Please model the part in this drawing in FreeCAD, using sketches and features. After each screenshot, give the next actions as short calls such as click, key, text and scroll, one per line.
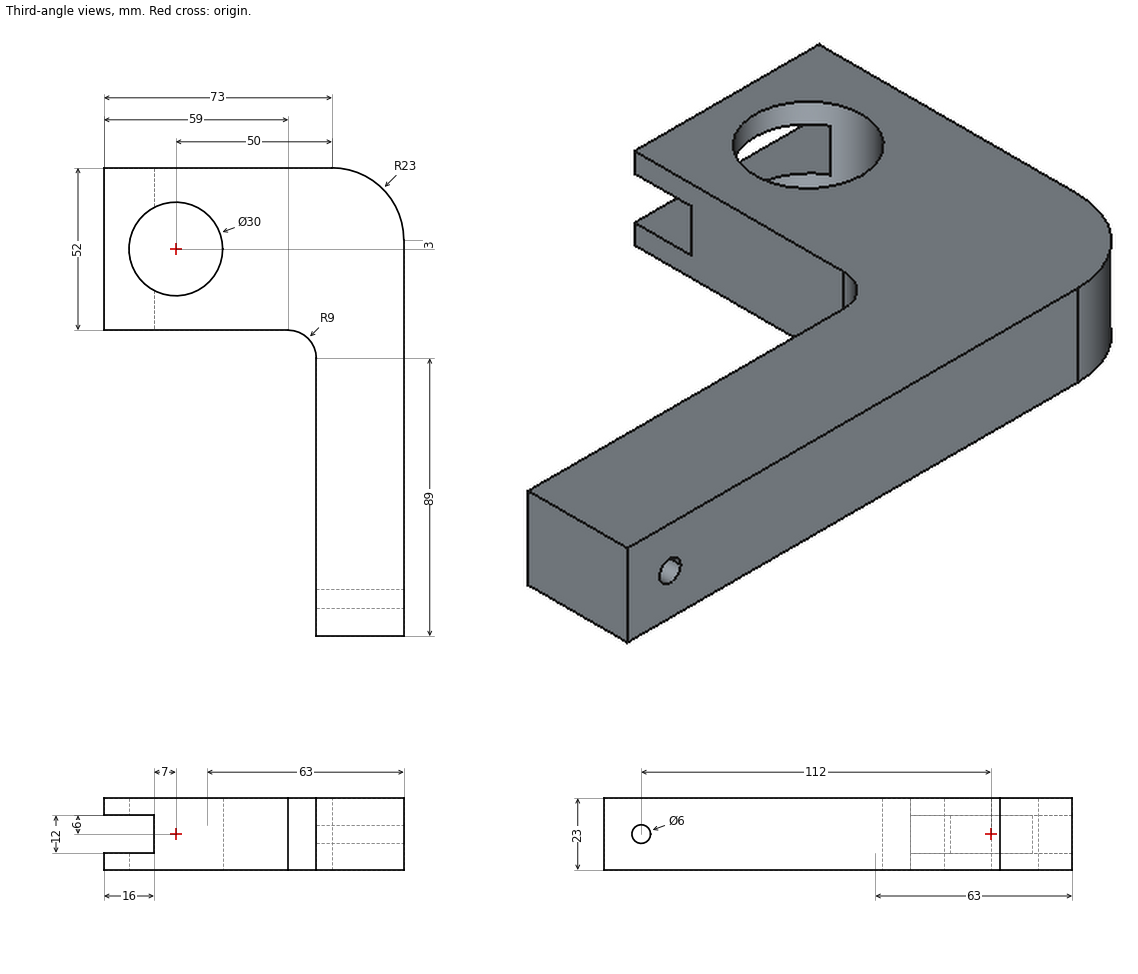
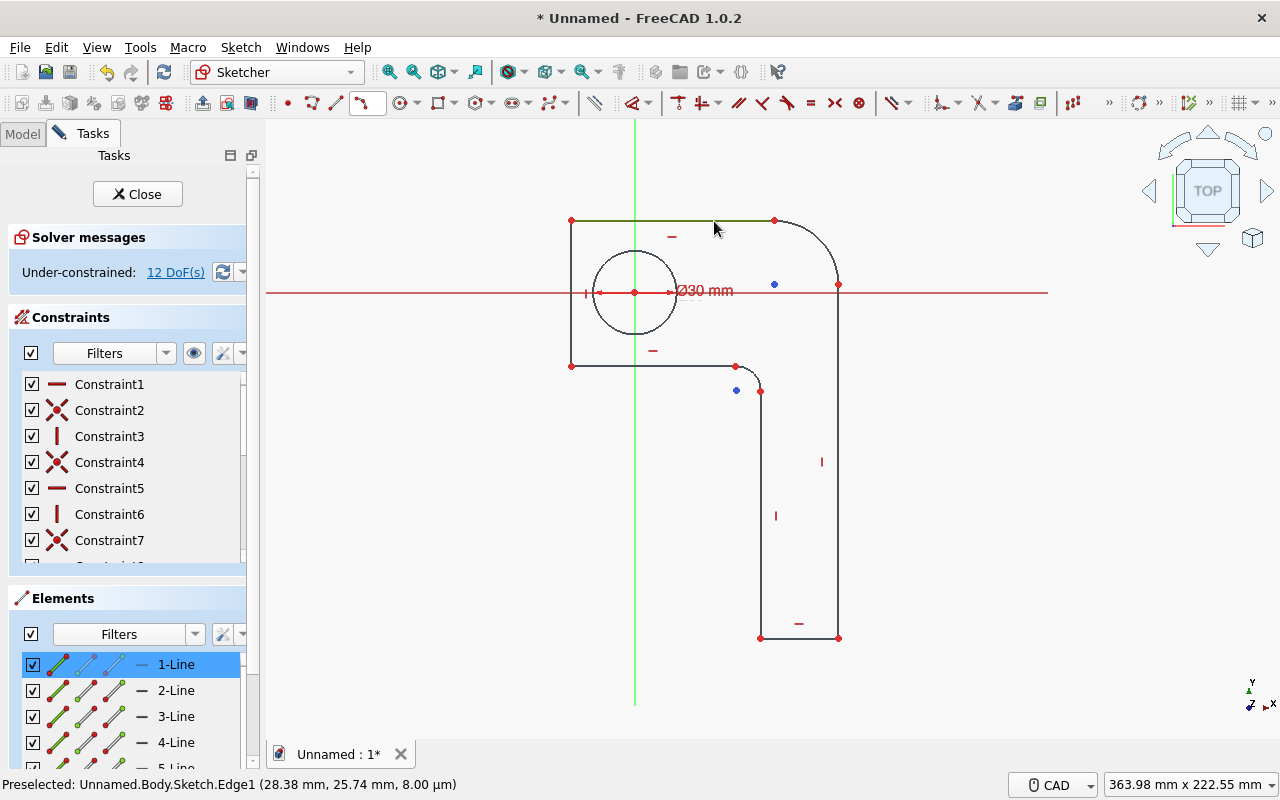
click(831, 256)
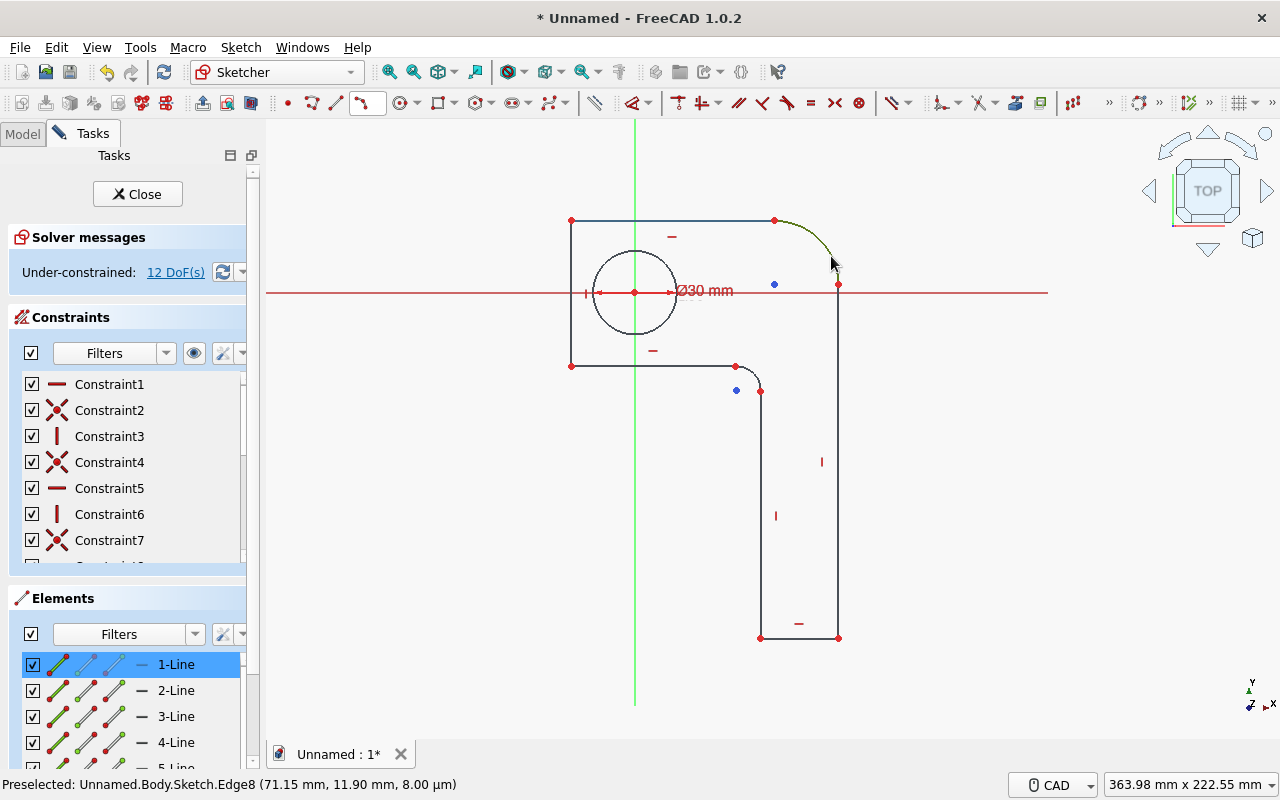
key(t)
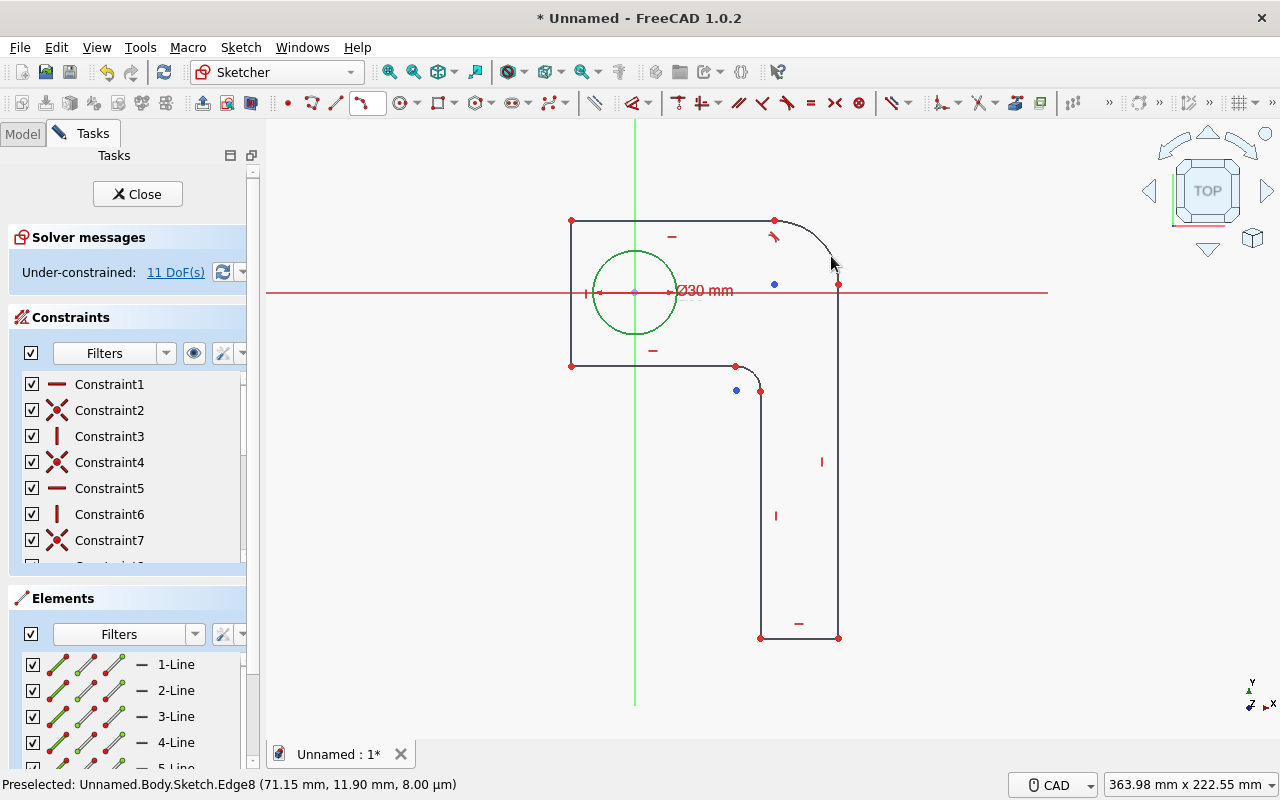
click(621, 366)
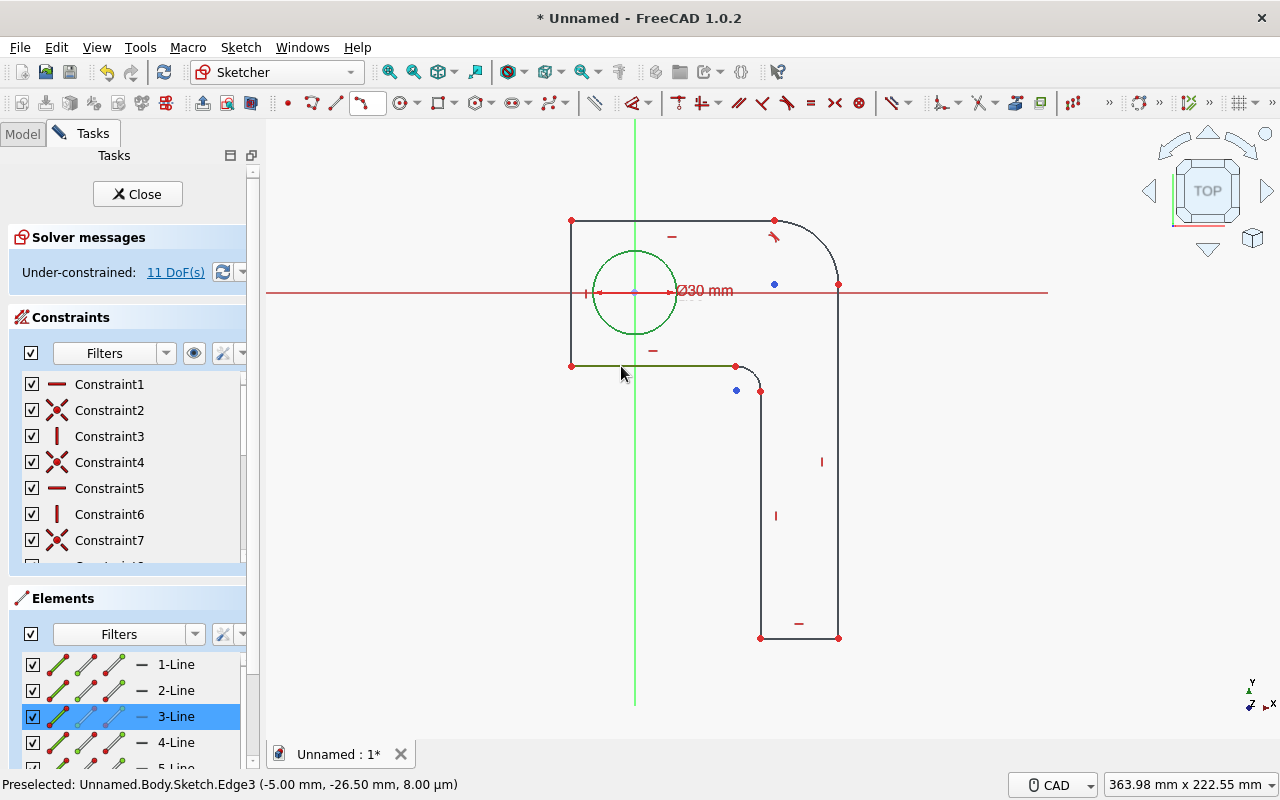
click(758, 380)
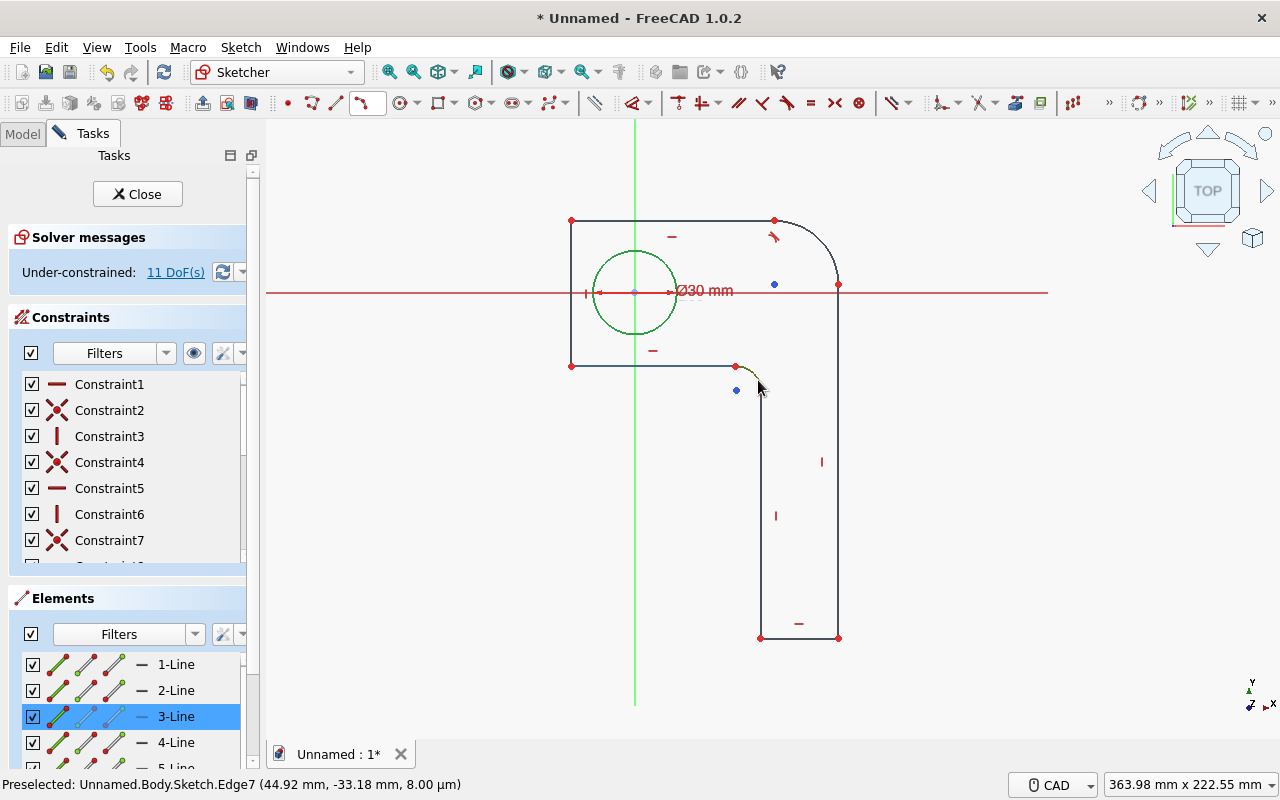
click(788, 104)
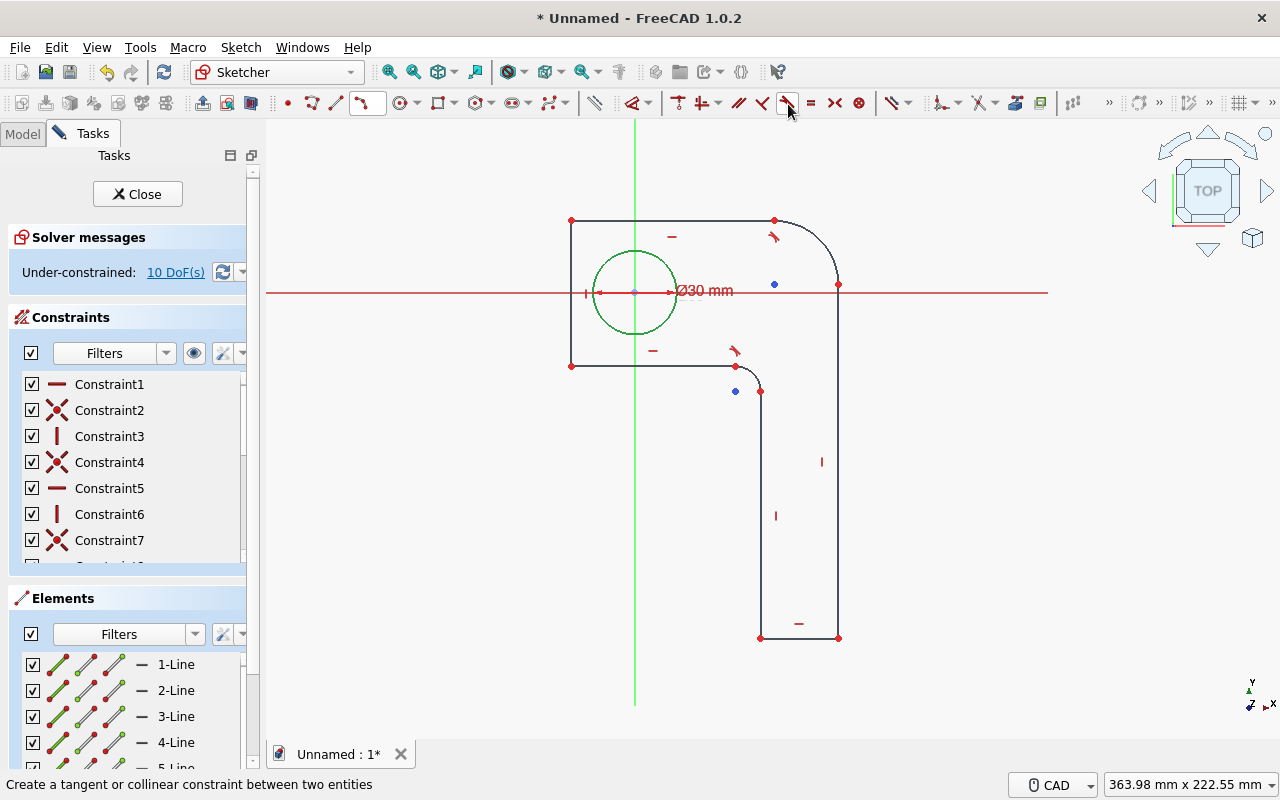
click(761, 466)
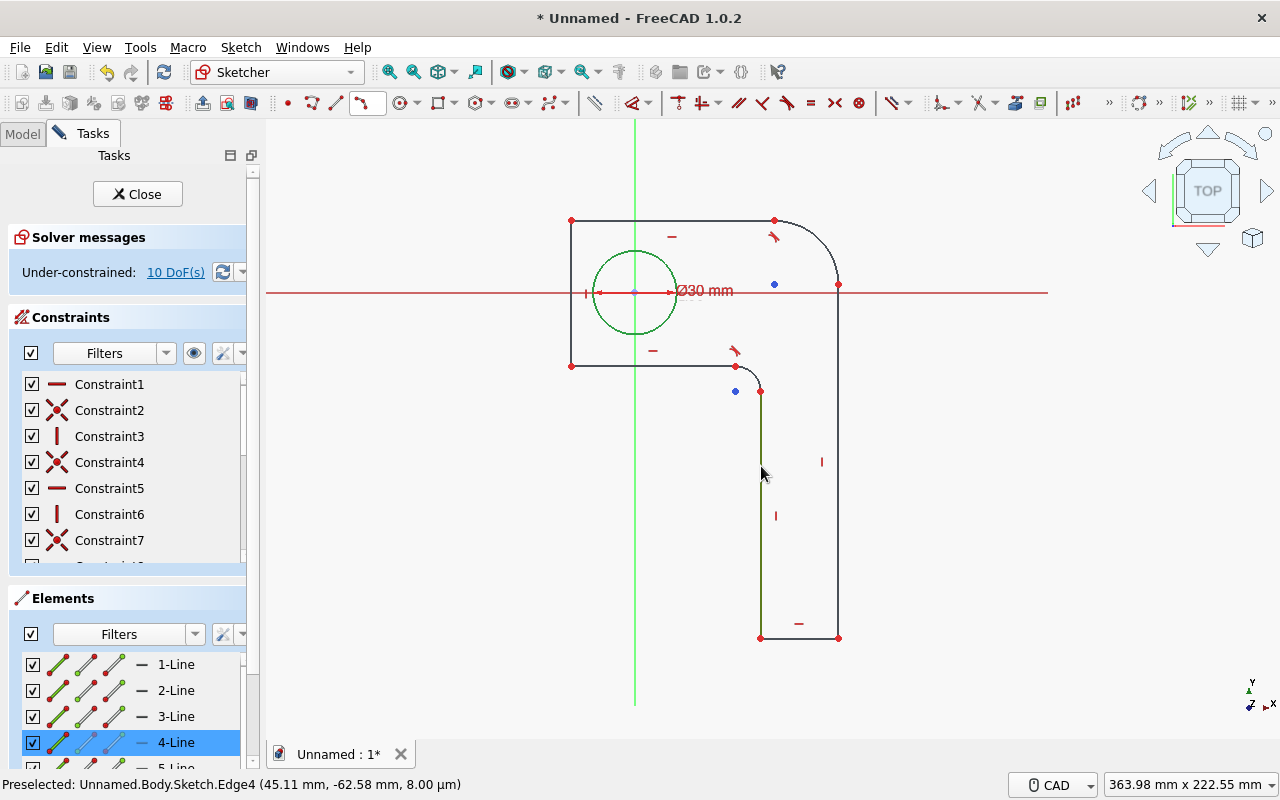
click(758, 380)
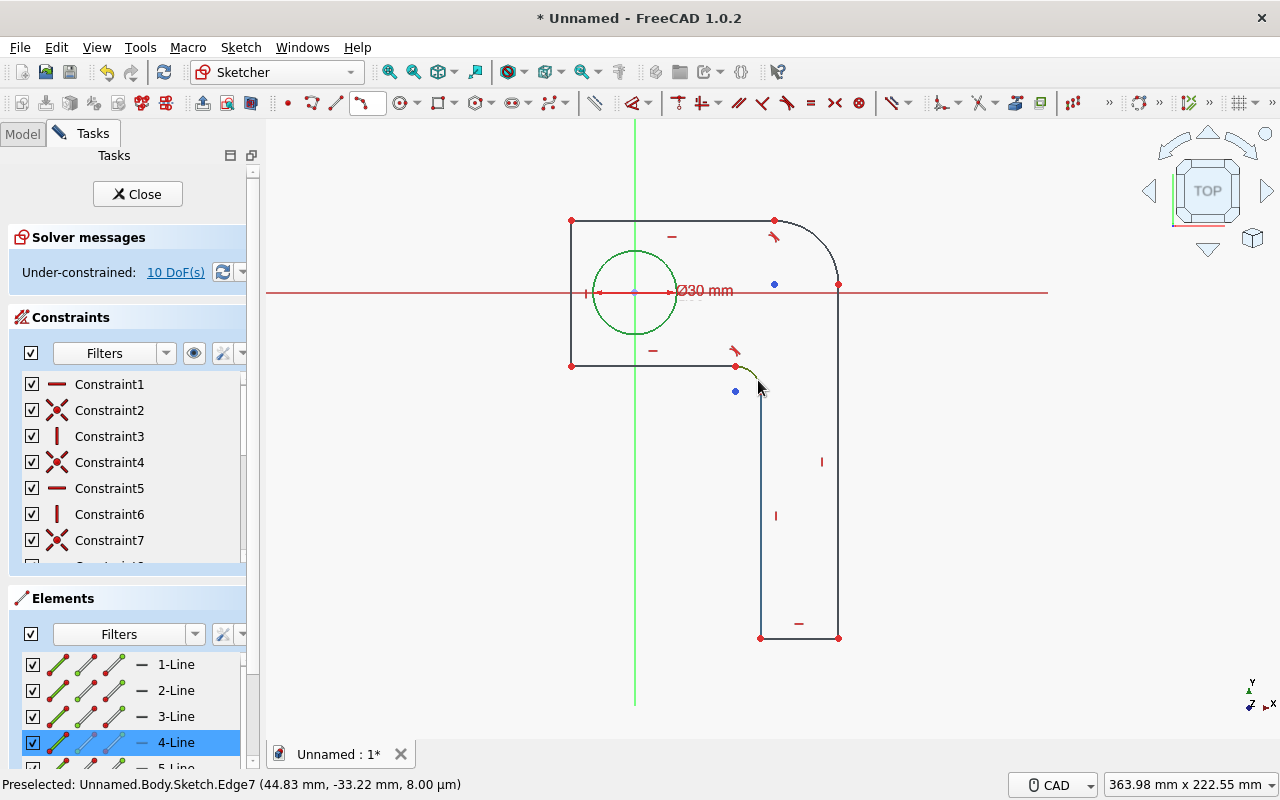
key(t)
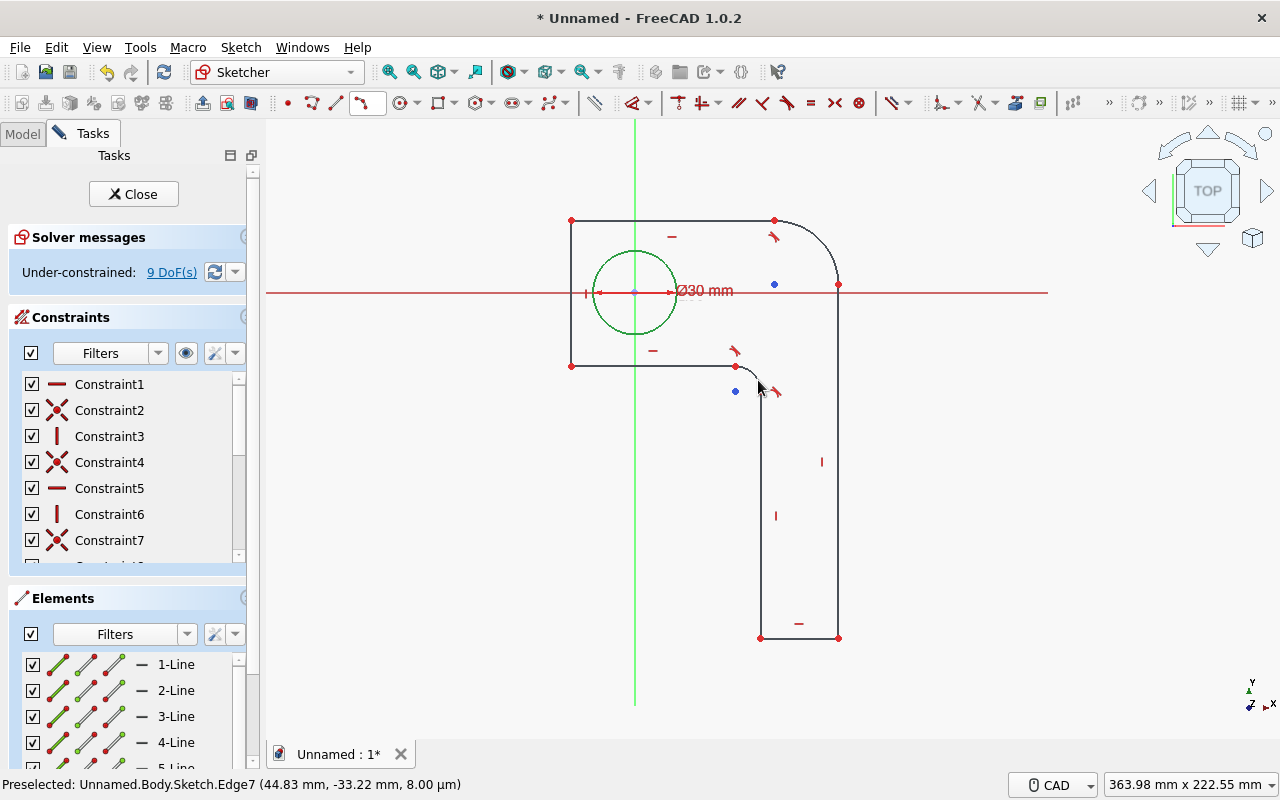
click(838, 533)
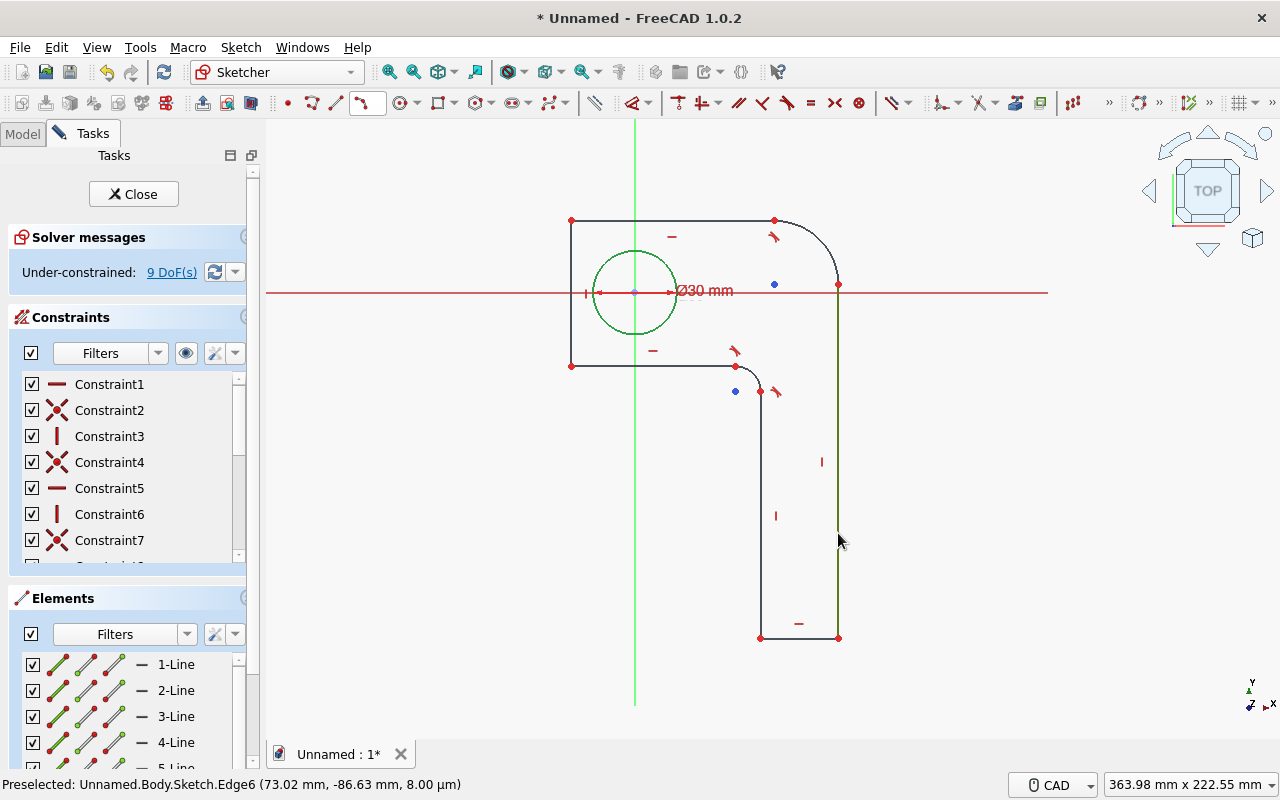
click(831, 256)